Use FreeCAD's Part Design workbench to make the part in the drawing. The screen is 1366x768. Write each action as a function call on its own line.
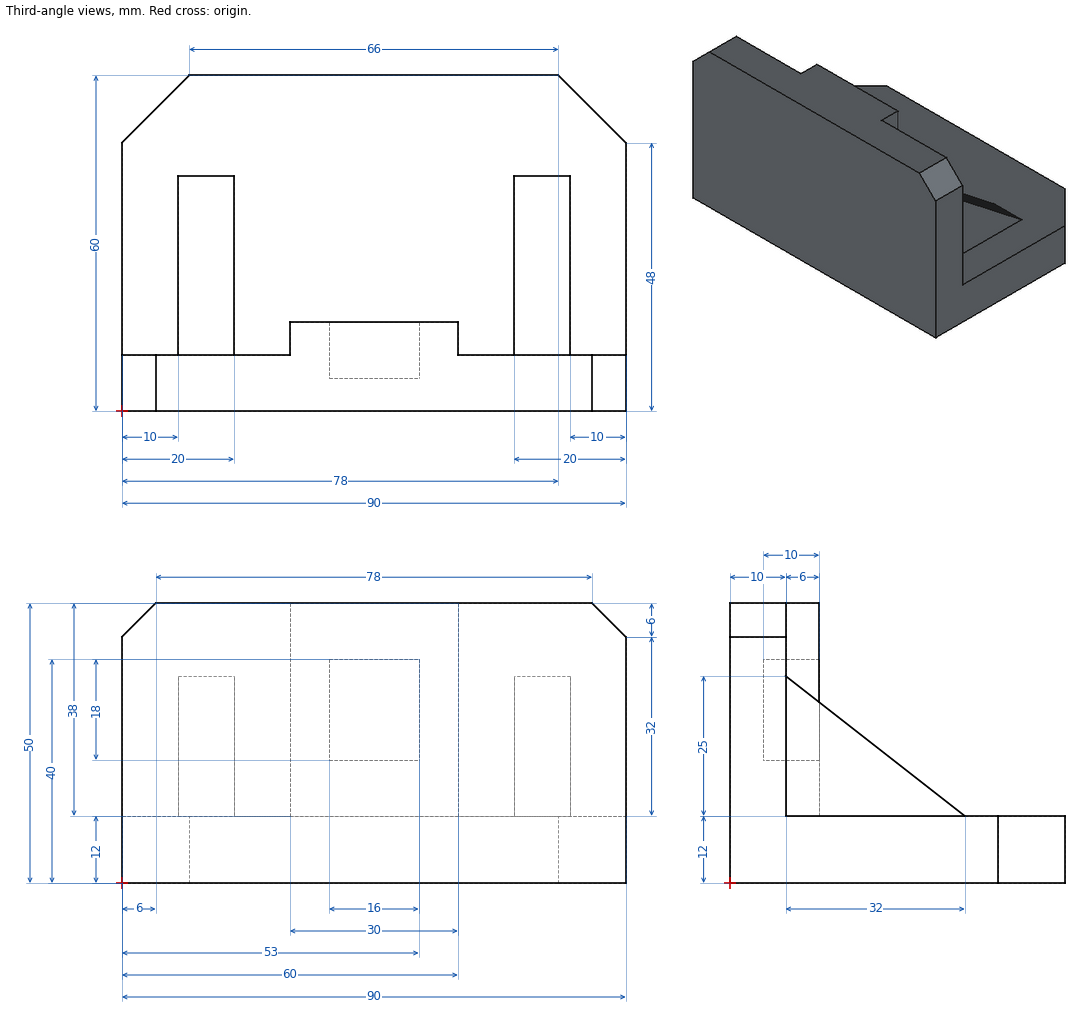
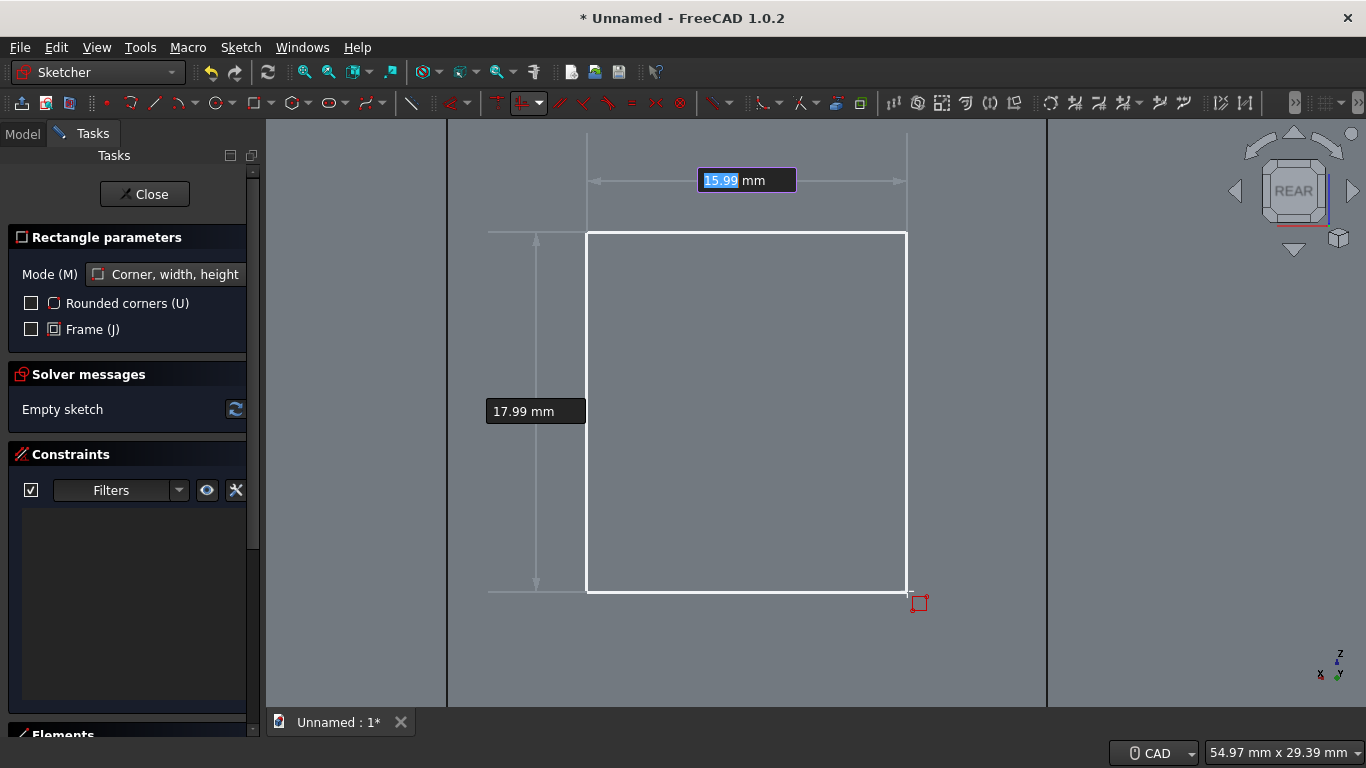
text(16)
key(Tab)
text(18)
key(Return)
key(Escape)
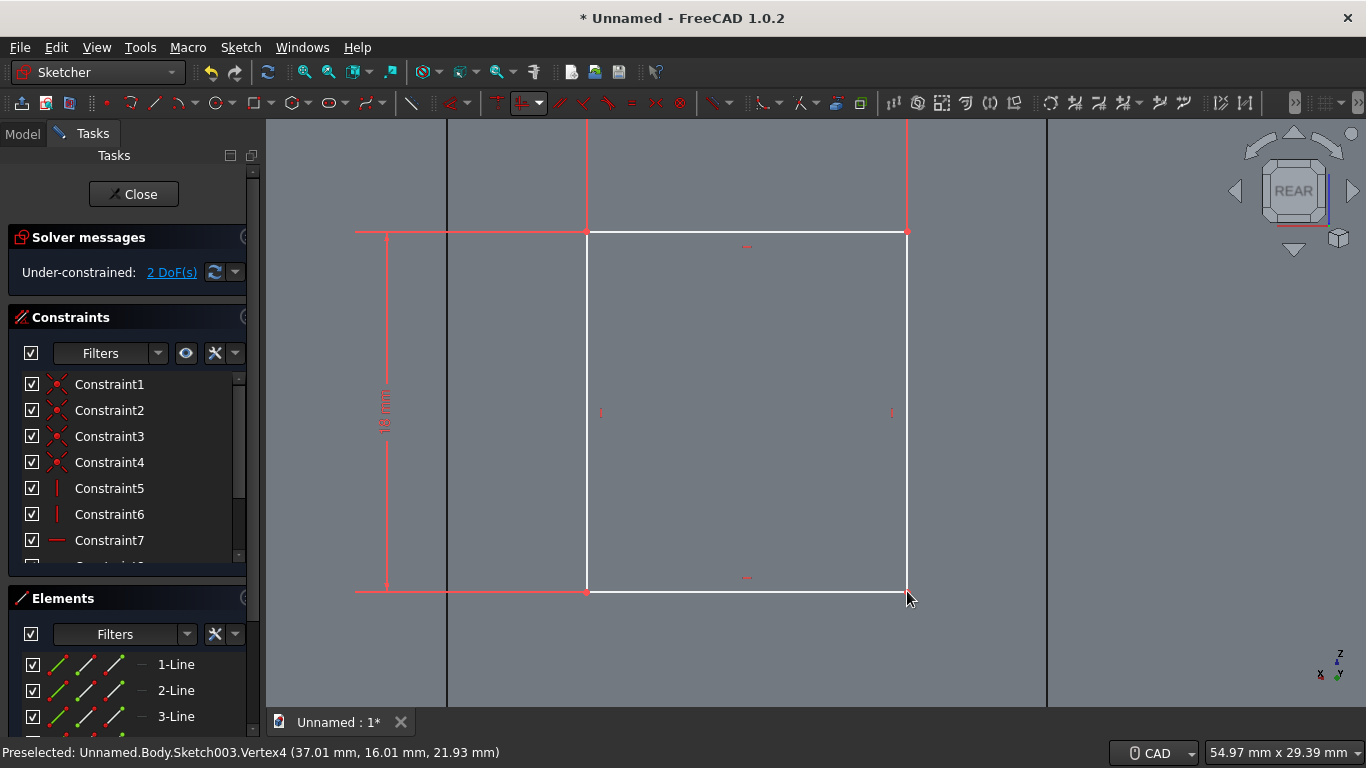
click(450, 104)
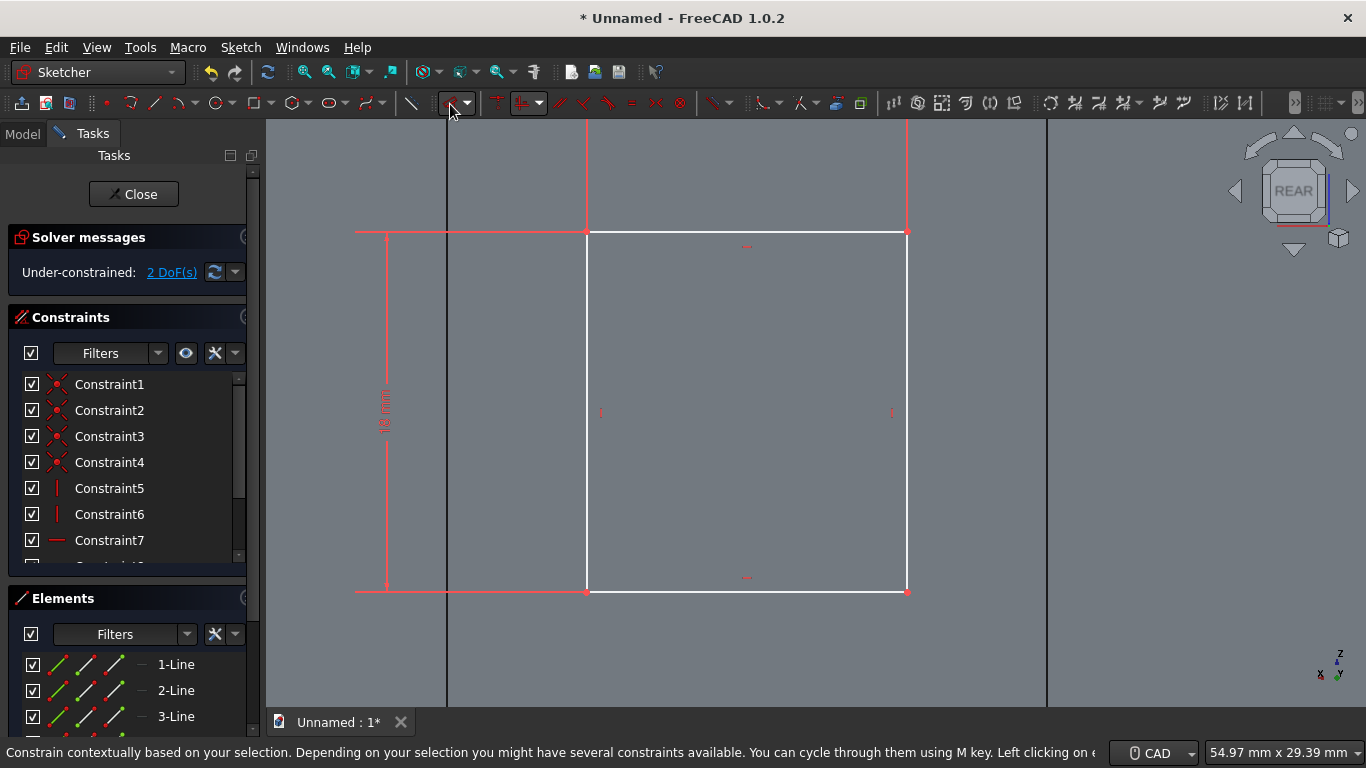
click(587, 232)
click(894, 198)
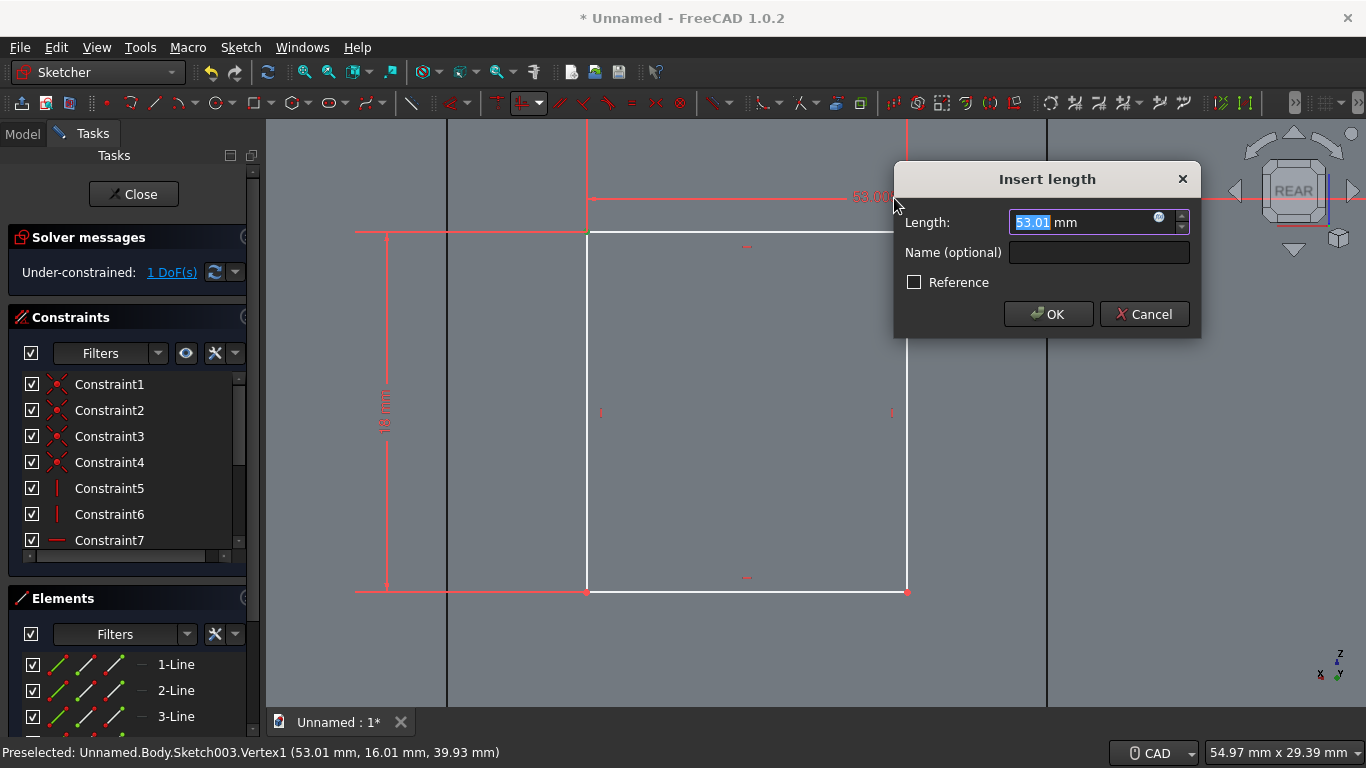
text(53)
key(Return)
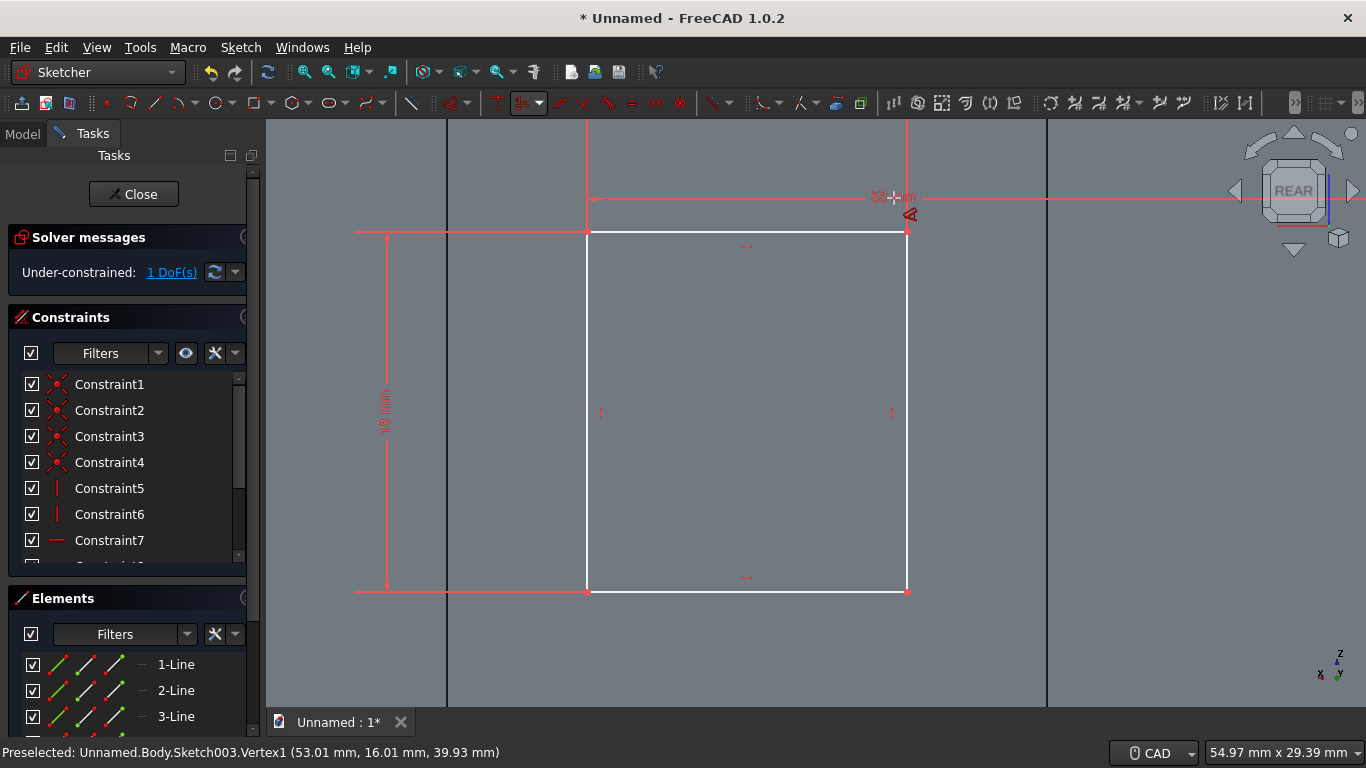
click(587, 232)
click(553, 455)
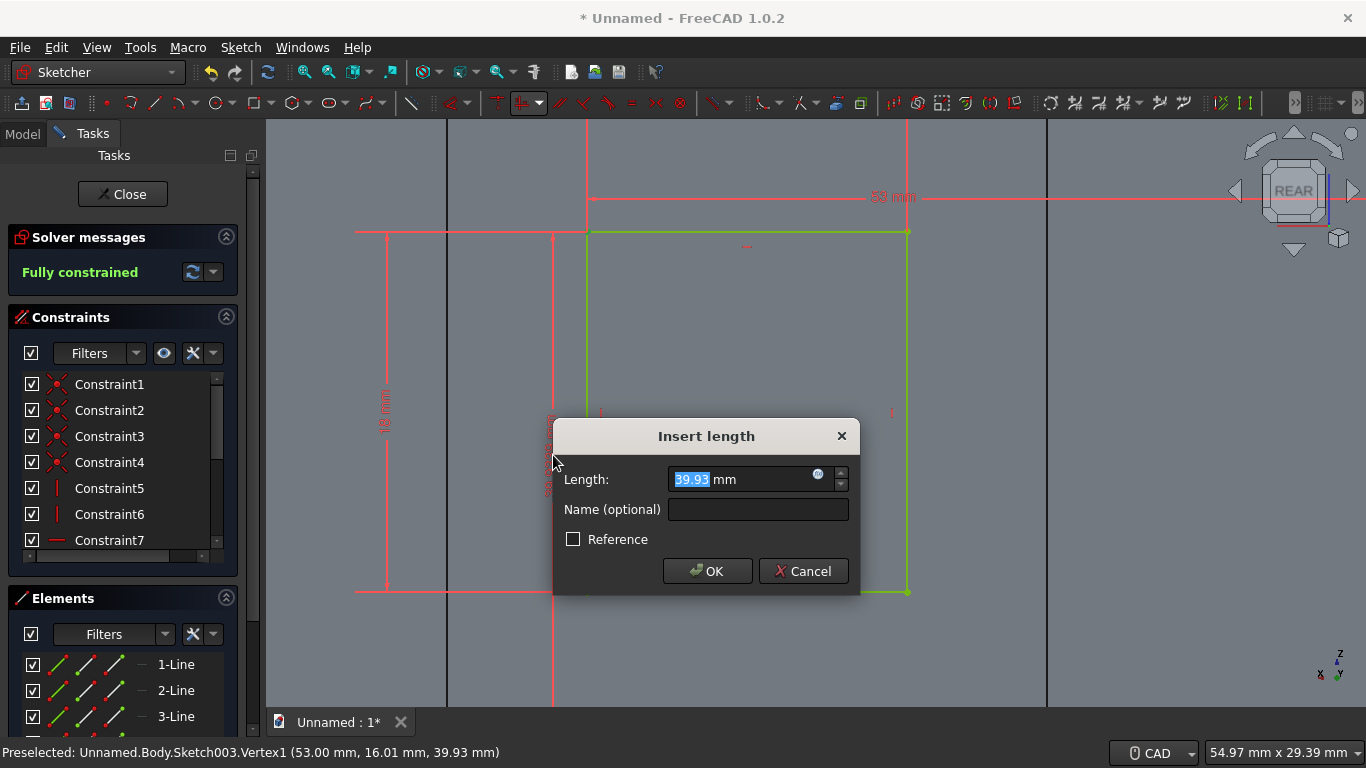
text(40)
key(Return)
key(Escape)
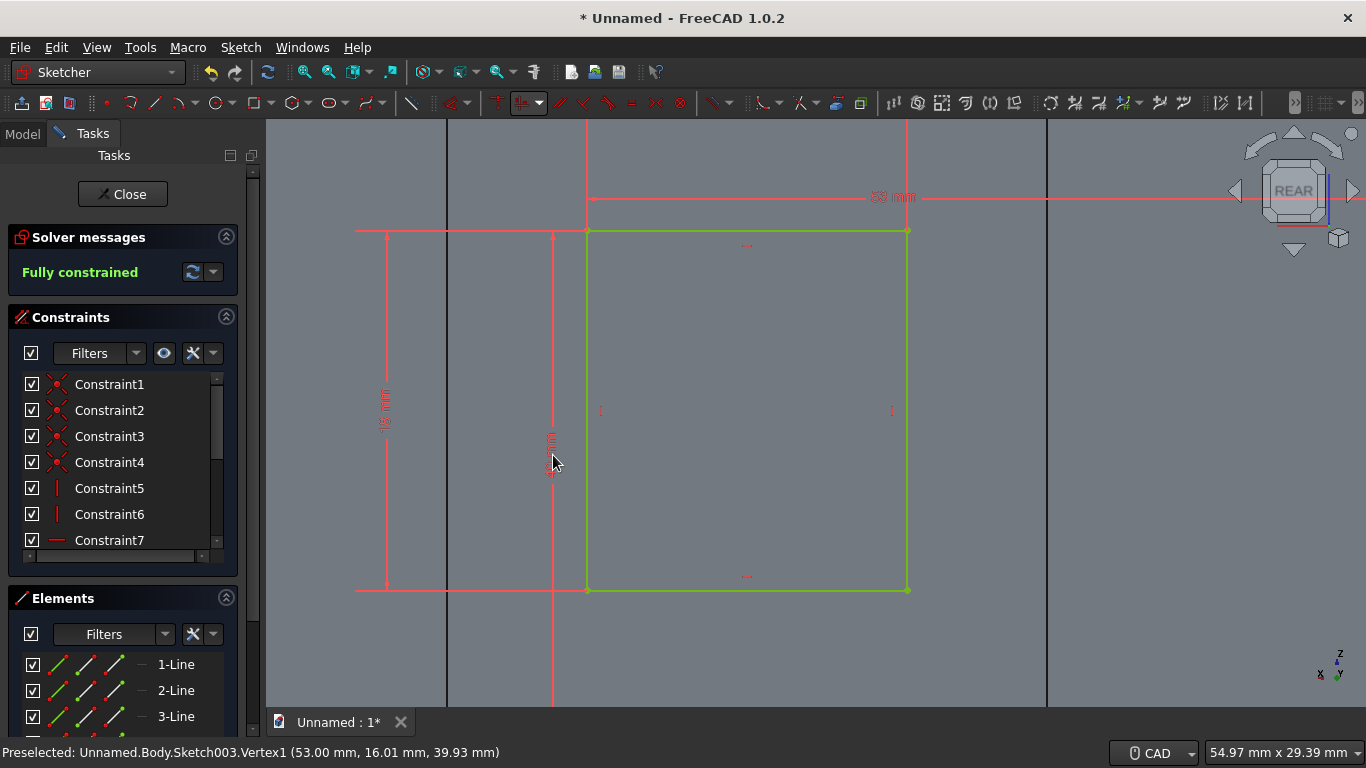
click(123, 194)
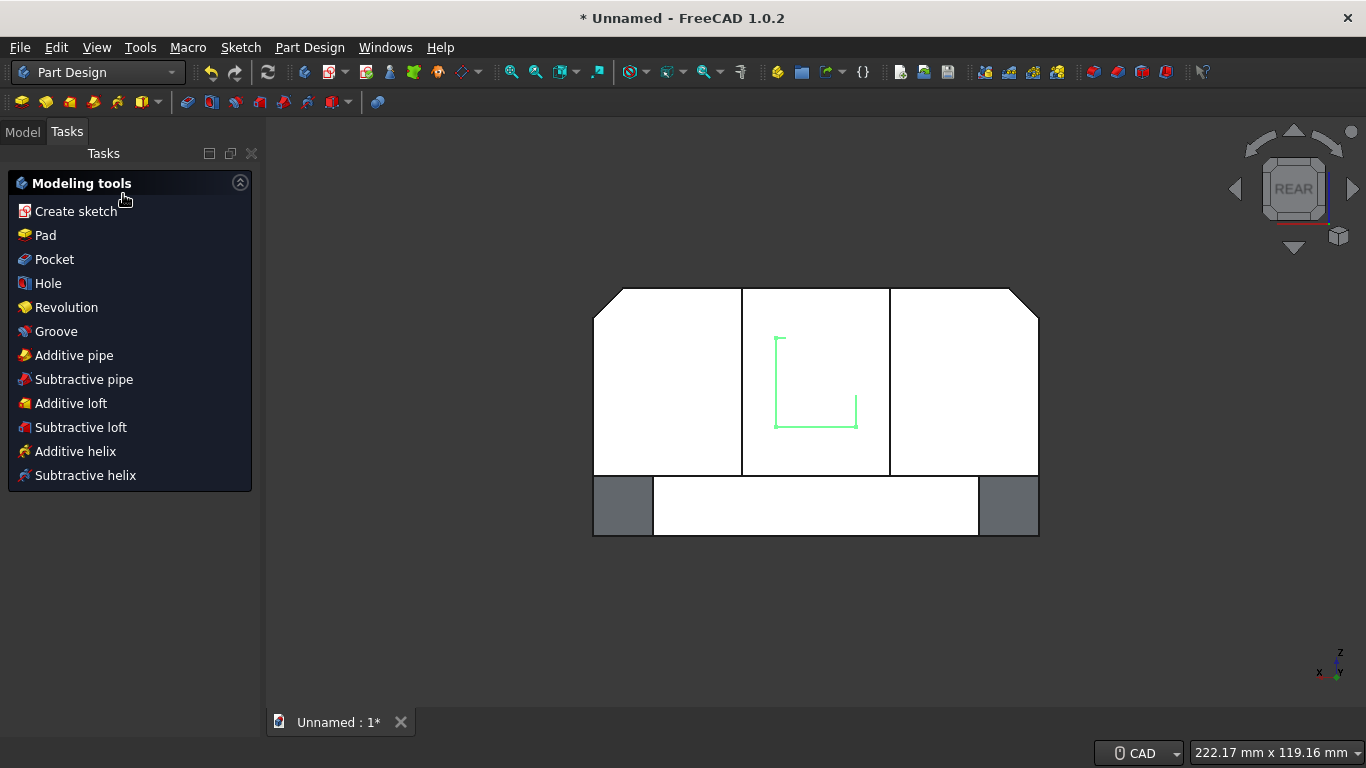
click(188, 102)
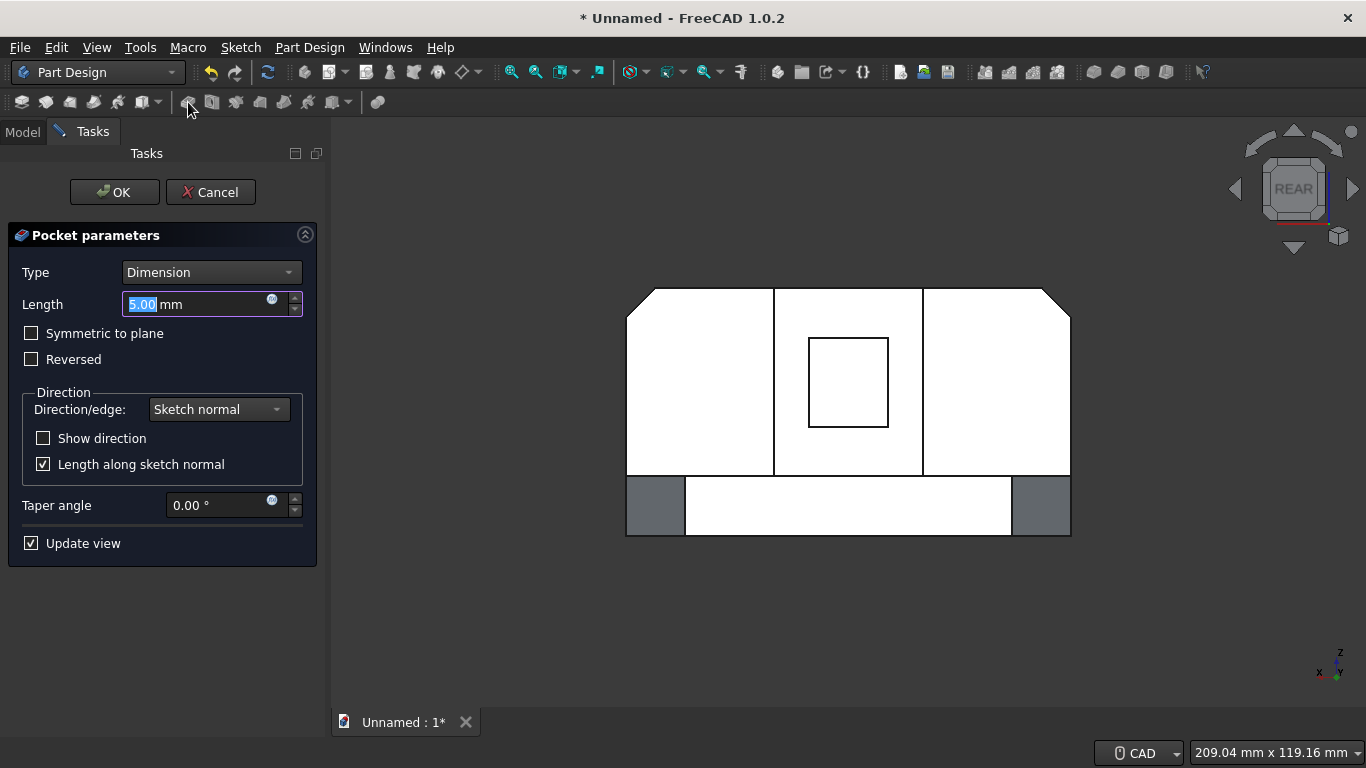
text(10)
key(Tab)